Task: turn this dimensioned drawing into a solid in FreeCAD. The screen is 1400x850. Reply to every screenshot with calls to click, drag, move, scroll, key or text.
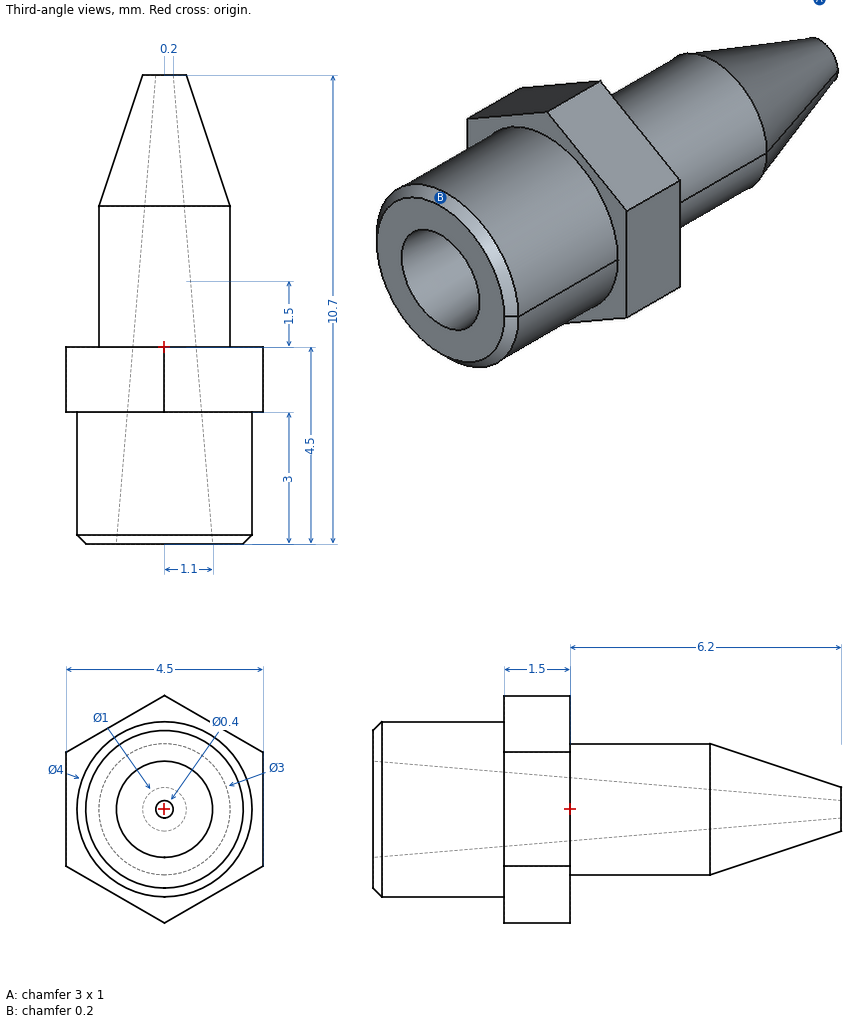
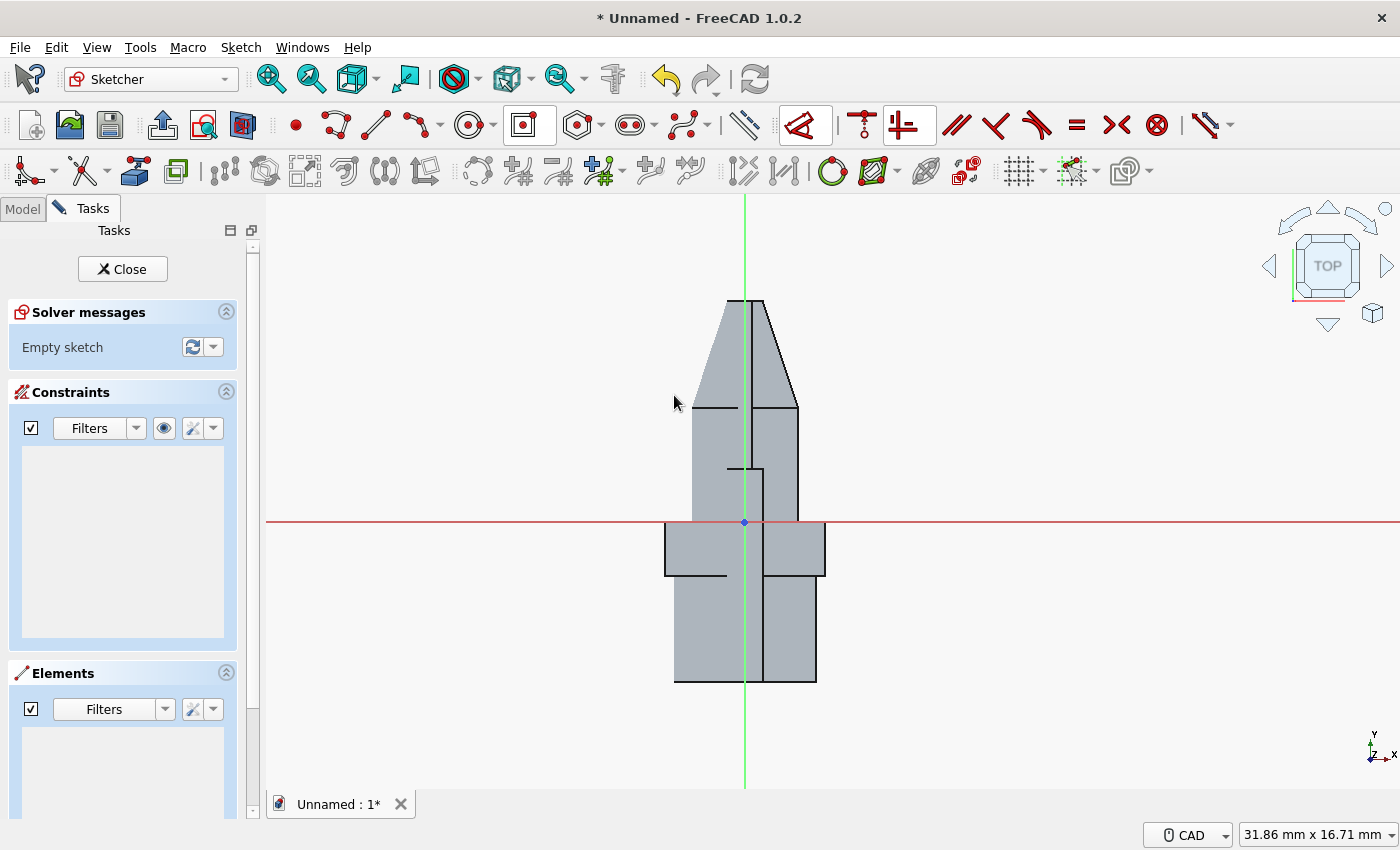
click(336, 126)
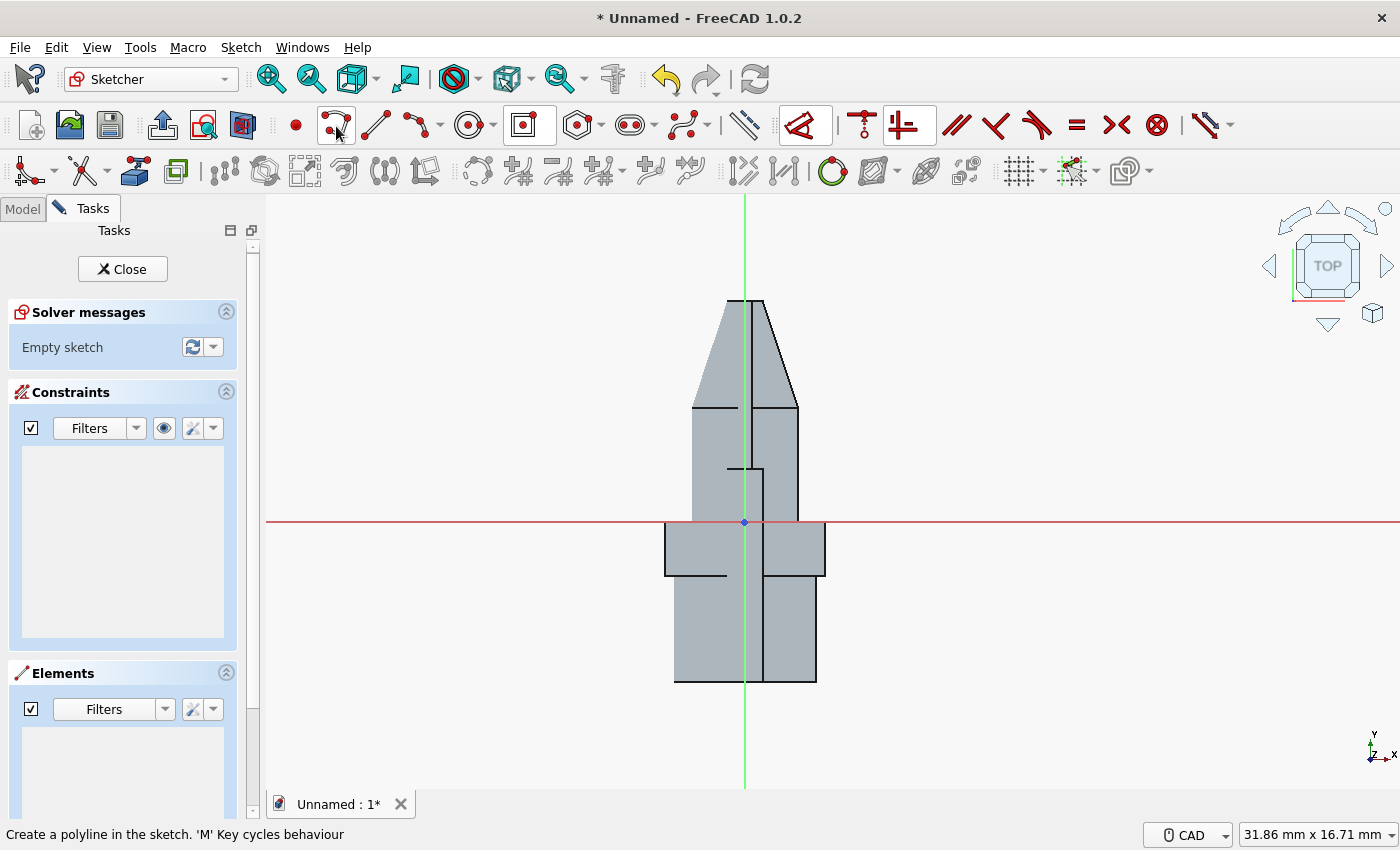
click(745, 682)
click(784, 682)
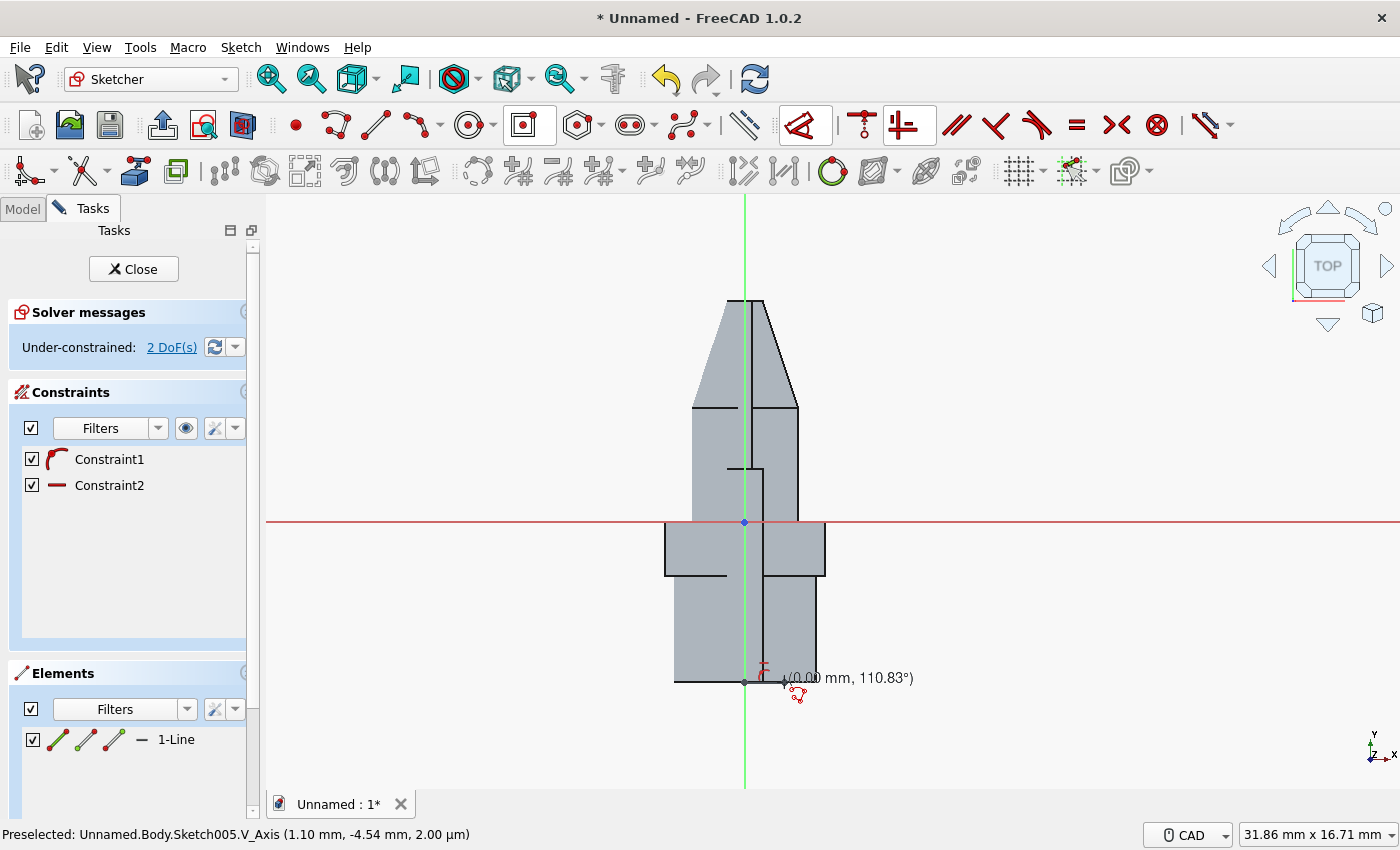
scroll(752, 301, up, 5)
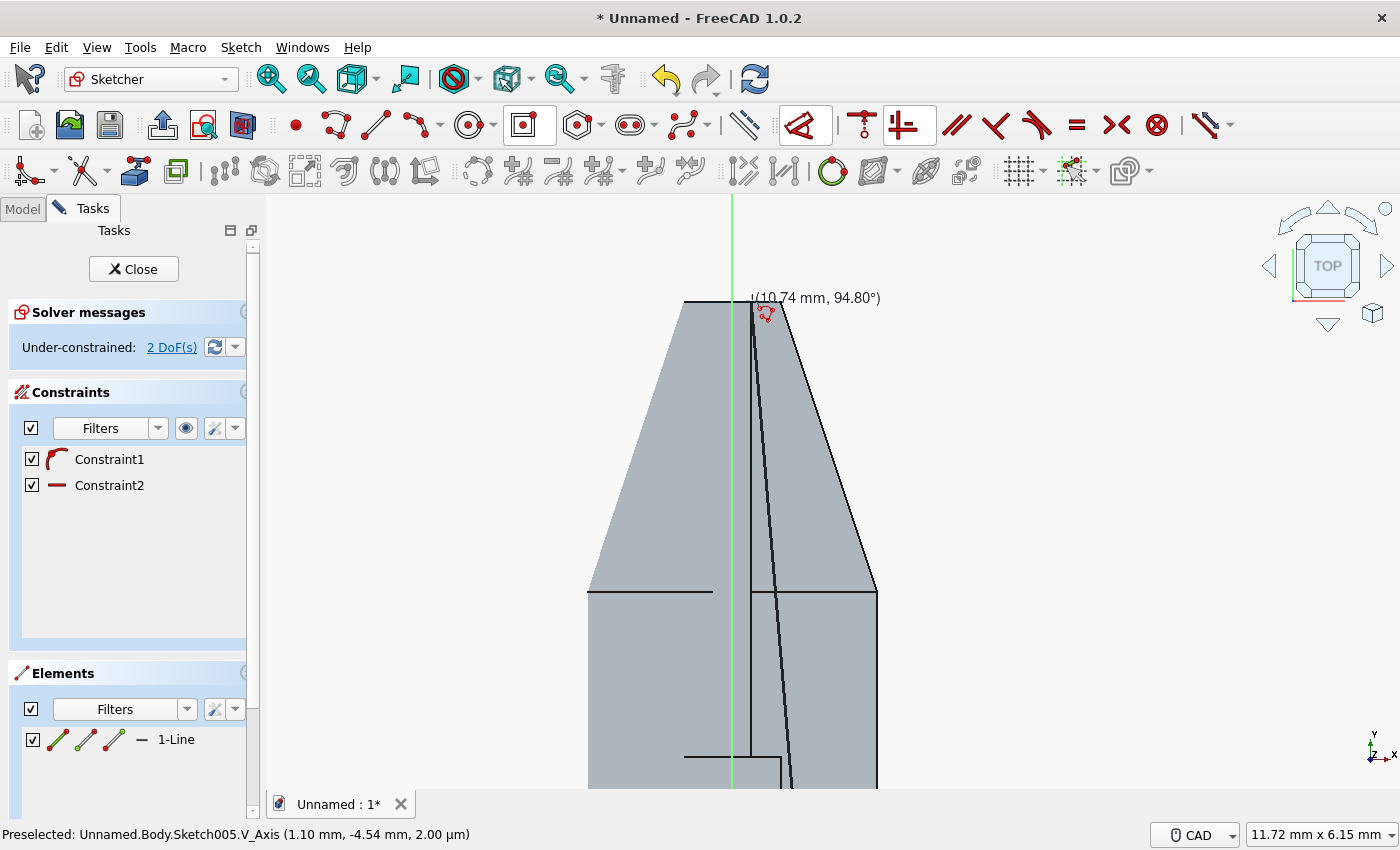
click(752, 302)
click(741, 302)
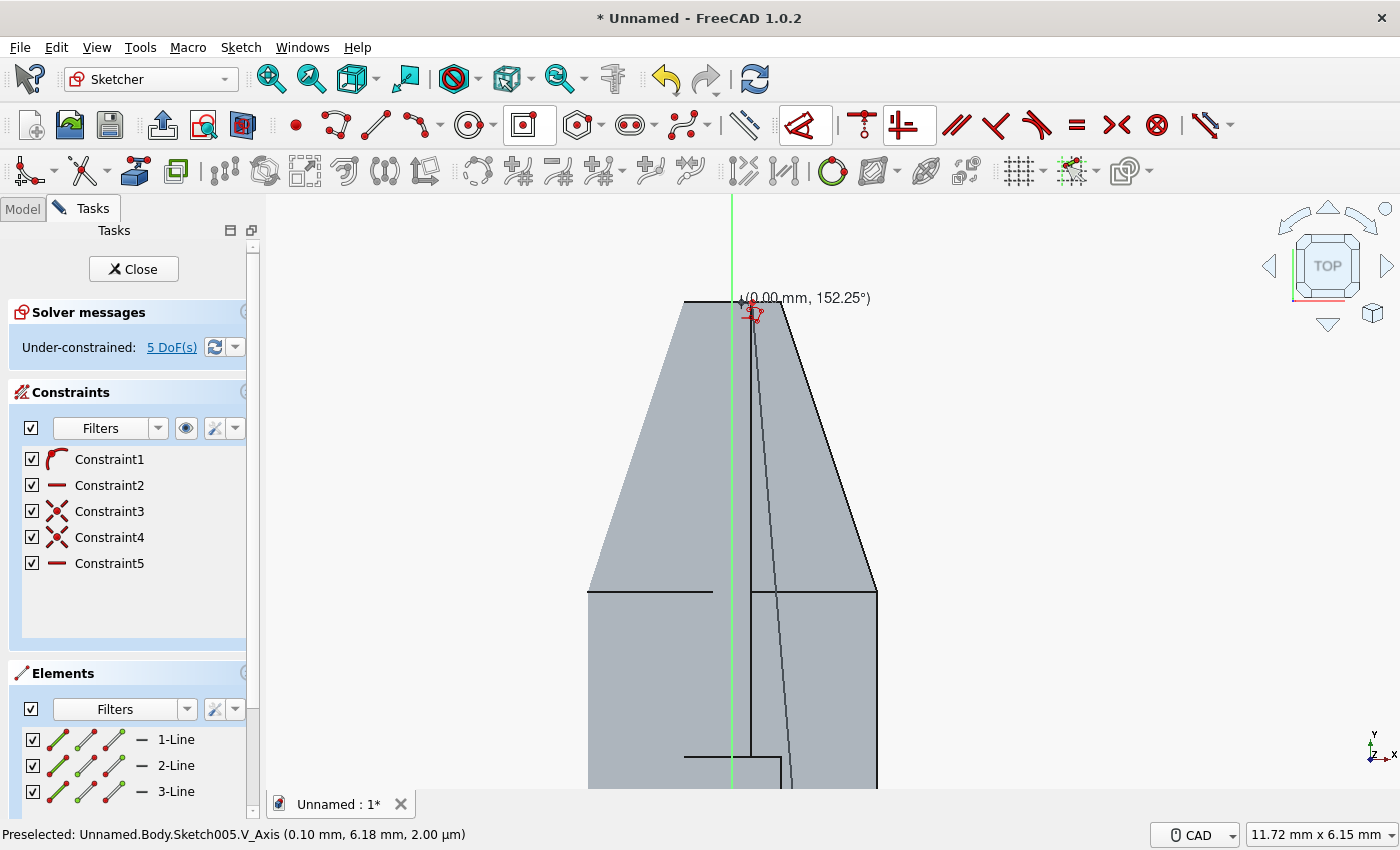
scroll(752, 300, down, 5)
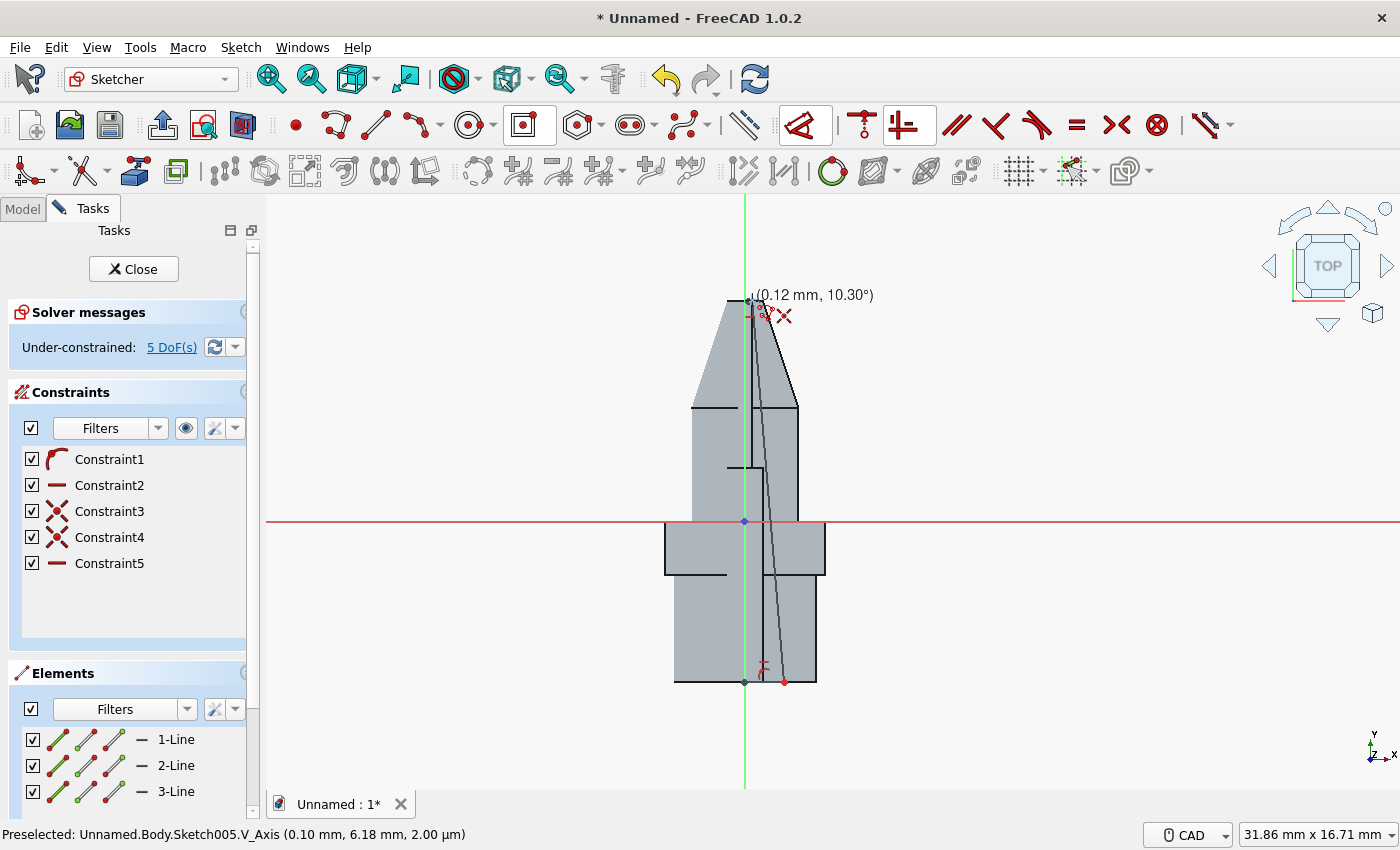
click(745, 682)
key(Escape)
key(Escape)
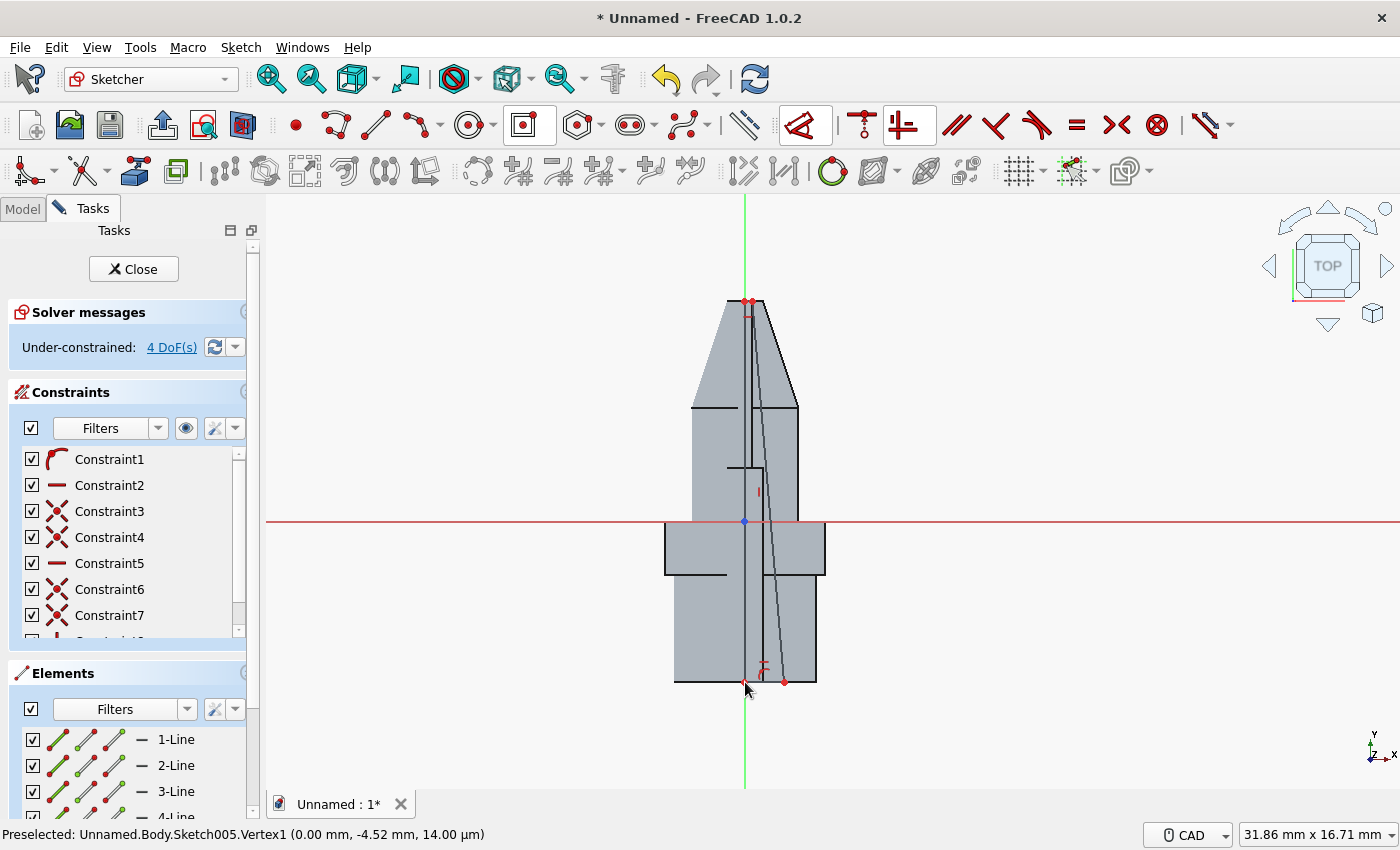
click(757, 682)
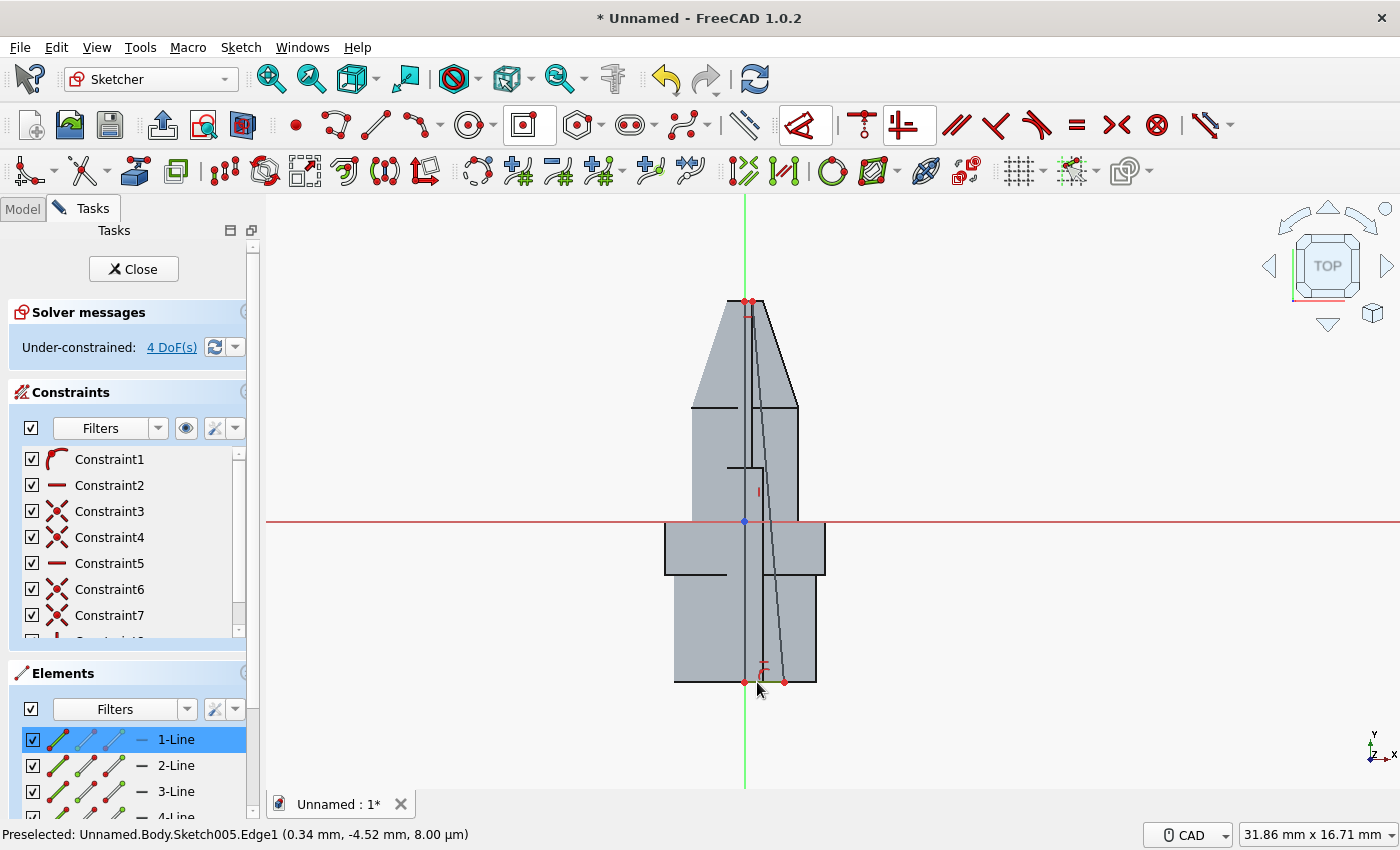
click(826, 126)